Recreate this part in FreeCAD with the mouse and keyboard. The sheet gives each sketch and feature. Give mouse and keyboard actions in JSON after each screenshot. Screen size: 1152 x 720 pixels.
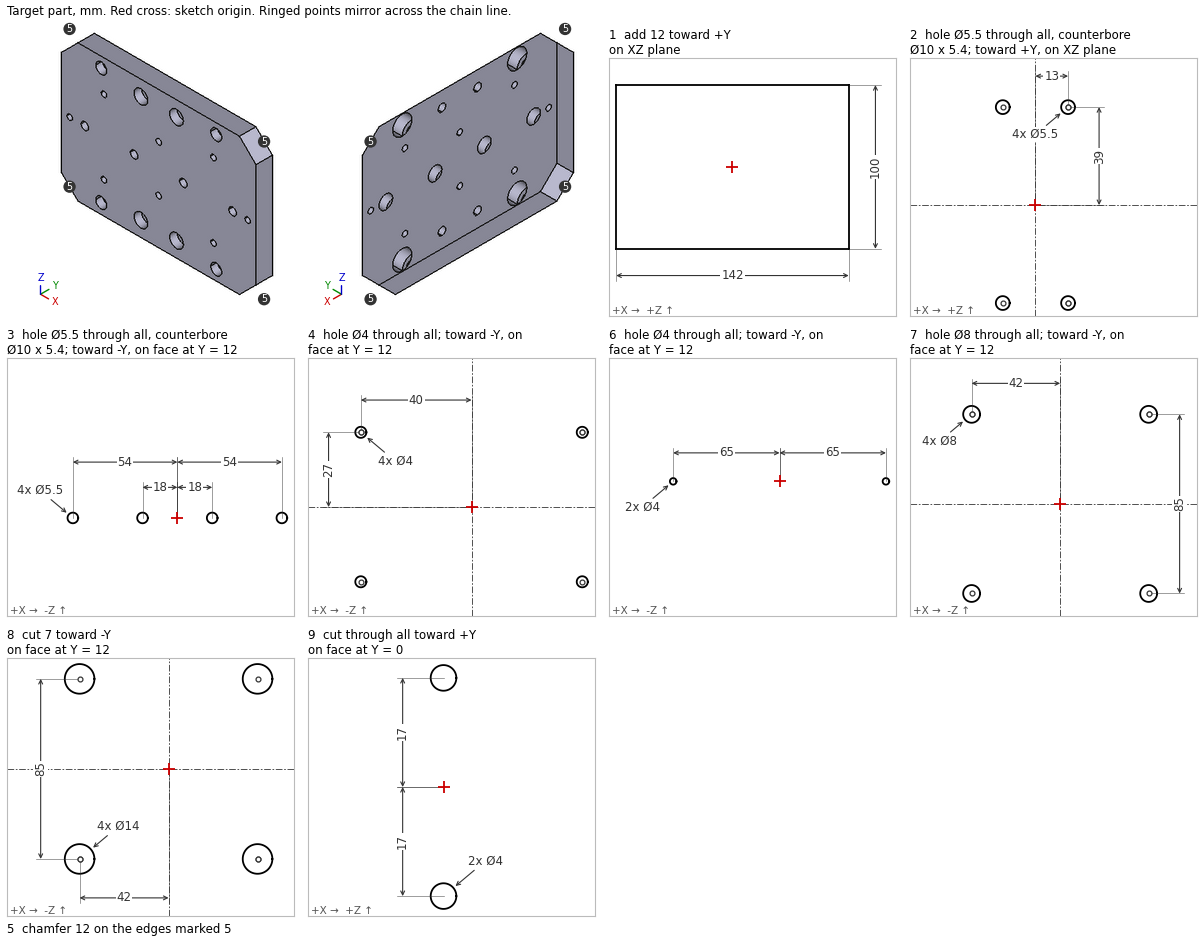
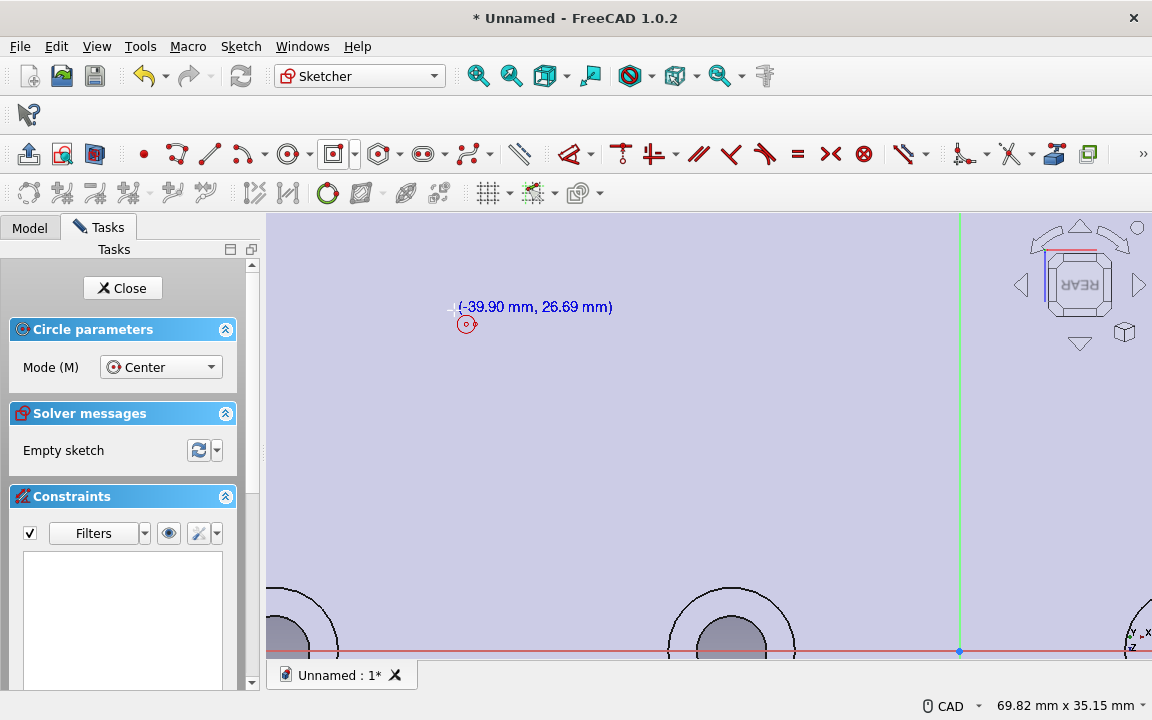
{"action": "left_click", "coordinate": [452, 308]}
{"action": "left_click", "coordinate": [470, 290]}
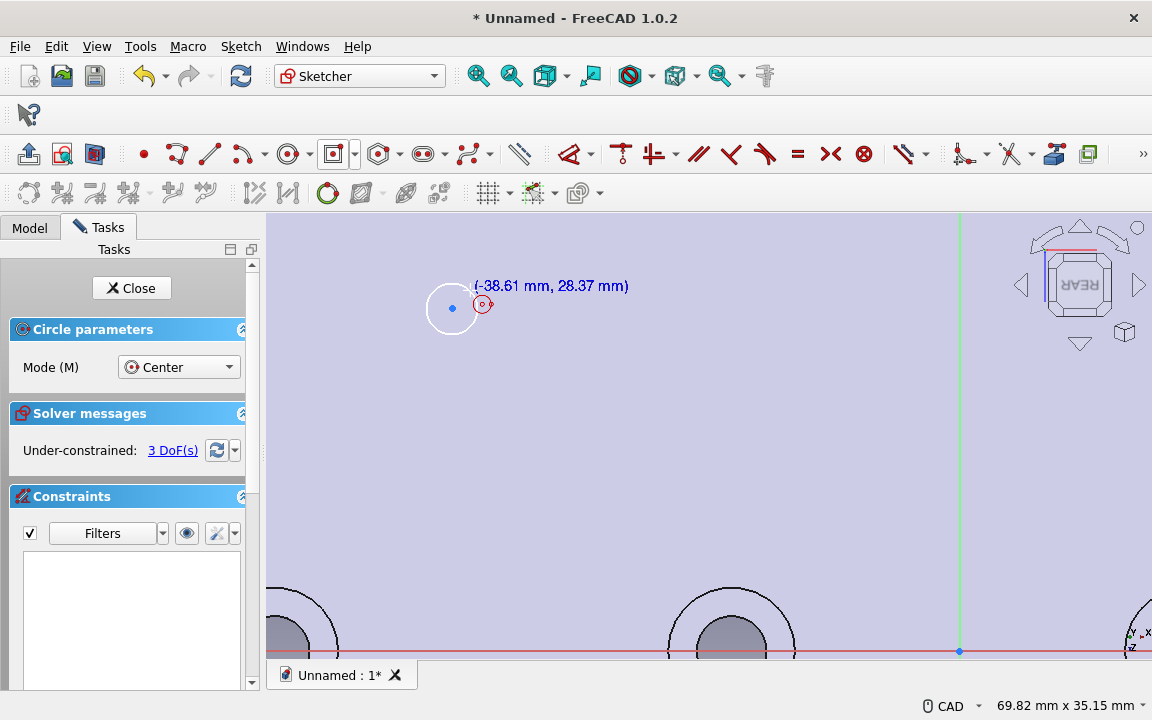
{"action": "scroll", "coordinate": [455, 311], "scroll_direction": "down", "scroll_amount": 5}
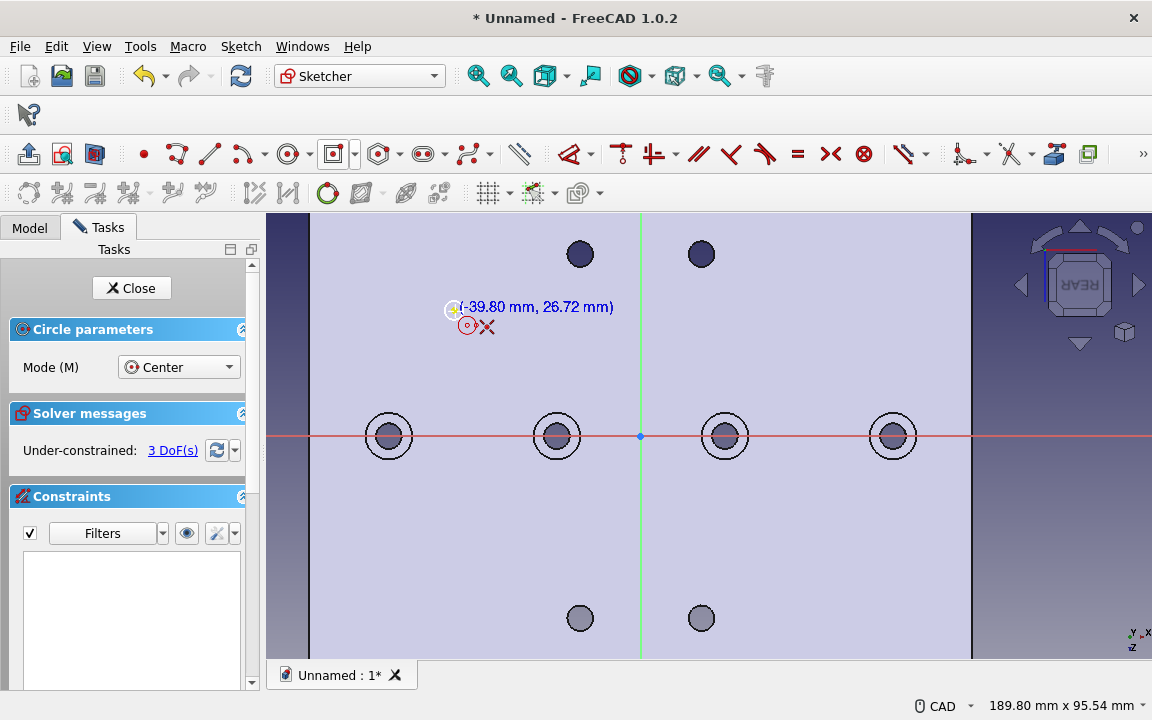
{"action": "scroll", "coordinate": [828, 310], "scroll_direction": "up", "scroll_amount": 5}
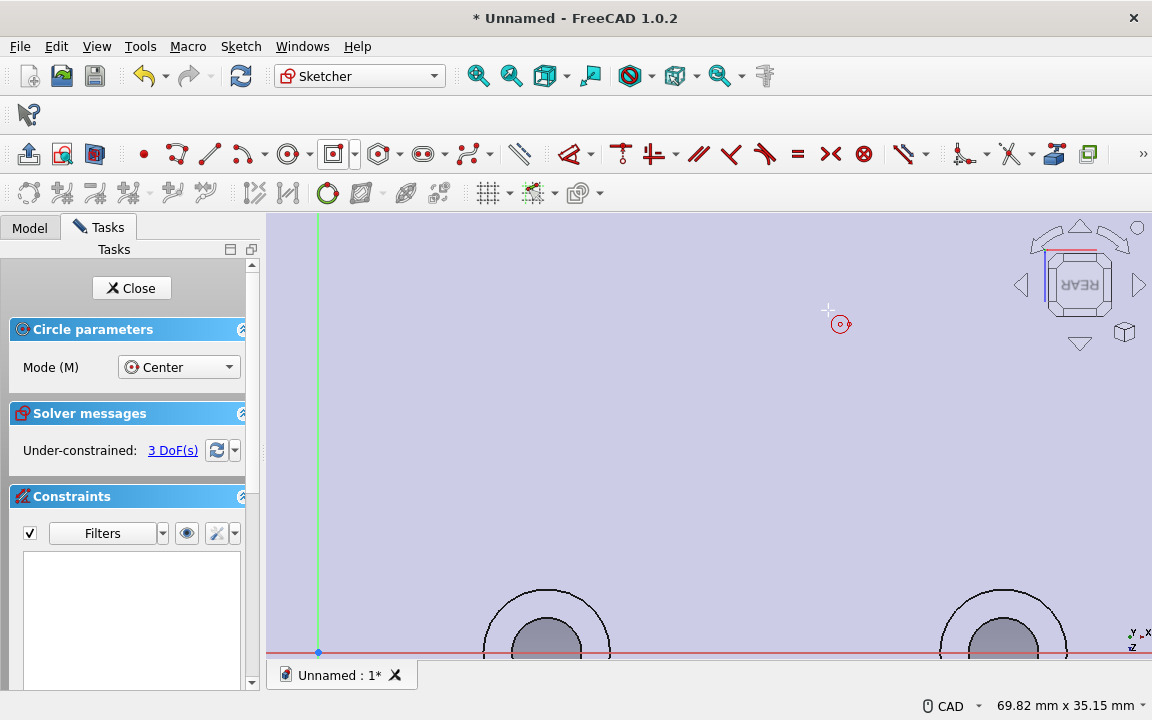
{"action": "left_click", "coordinate": [826, 310]}
{"action": "left_click", "coordinate": [844, 292]}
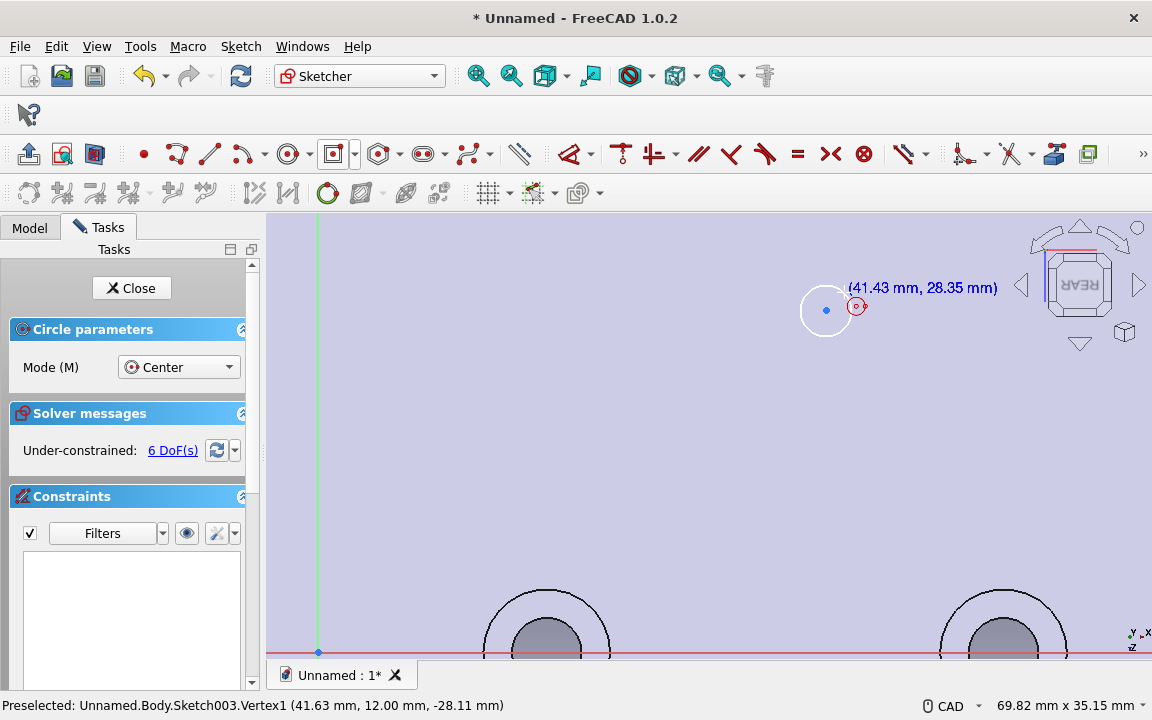
{"action": "scroll", "coordinate": [828, 310], "scroll_direction": "down", "scroll_amount": 5}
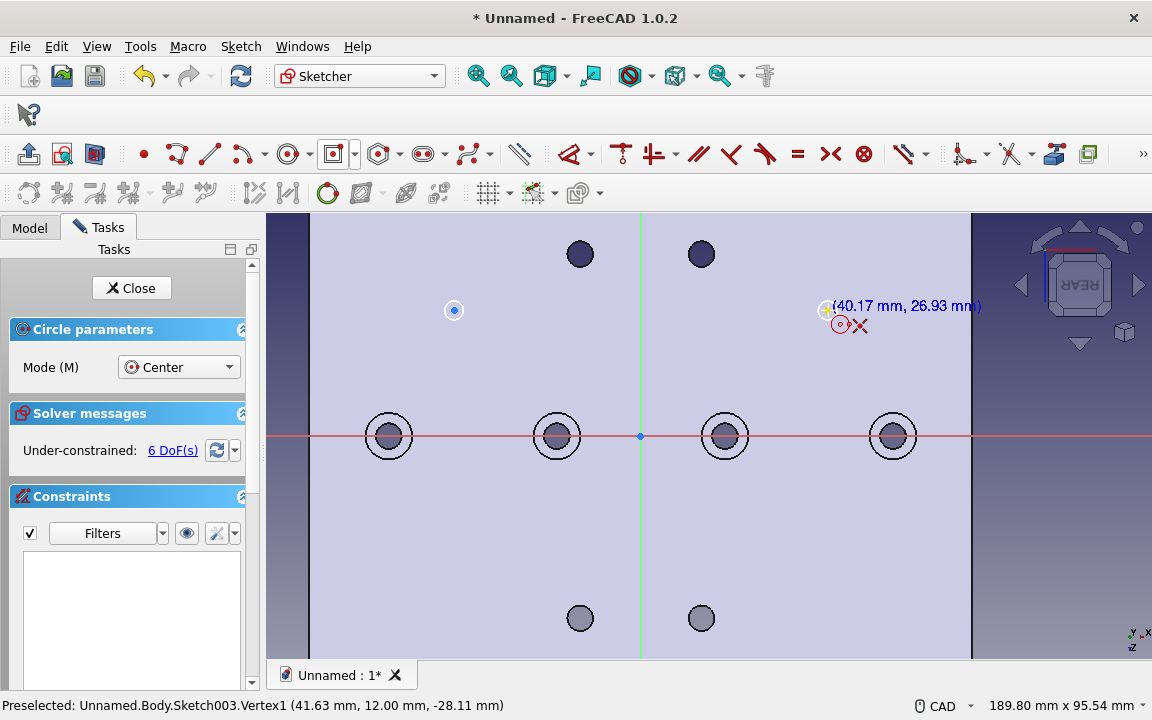
{"action": "scroll", "coordinate": [828, 562], "scroll_direction": "up", "scroll_amount": 5}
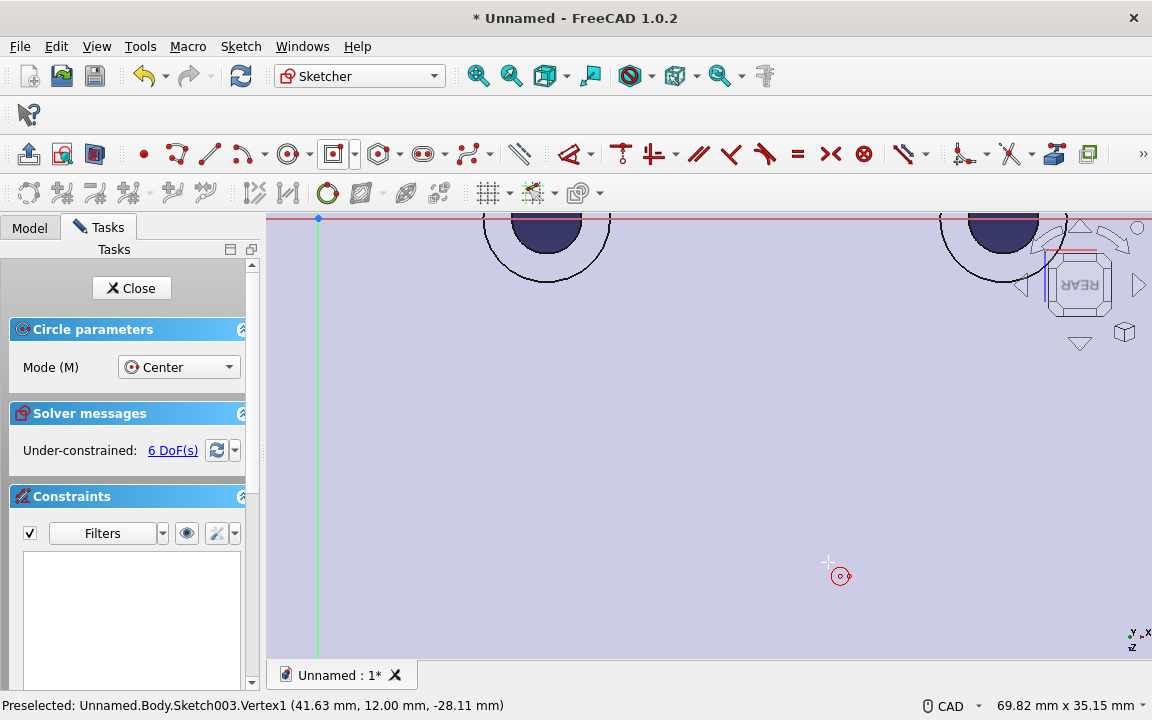
{"action": "left_click", "coordinate": [826, 561]}
{"action": "left_click", "coordinate": [844, 543]}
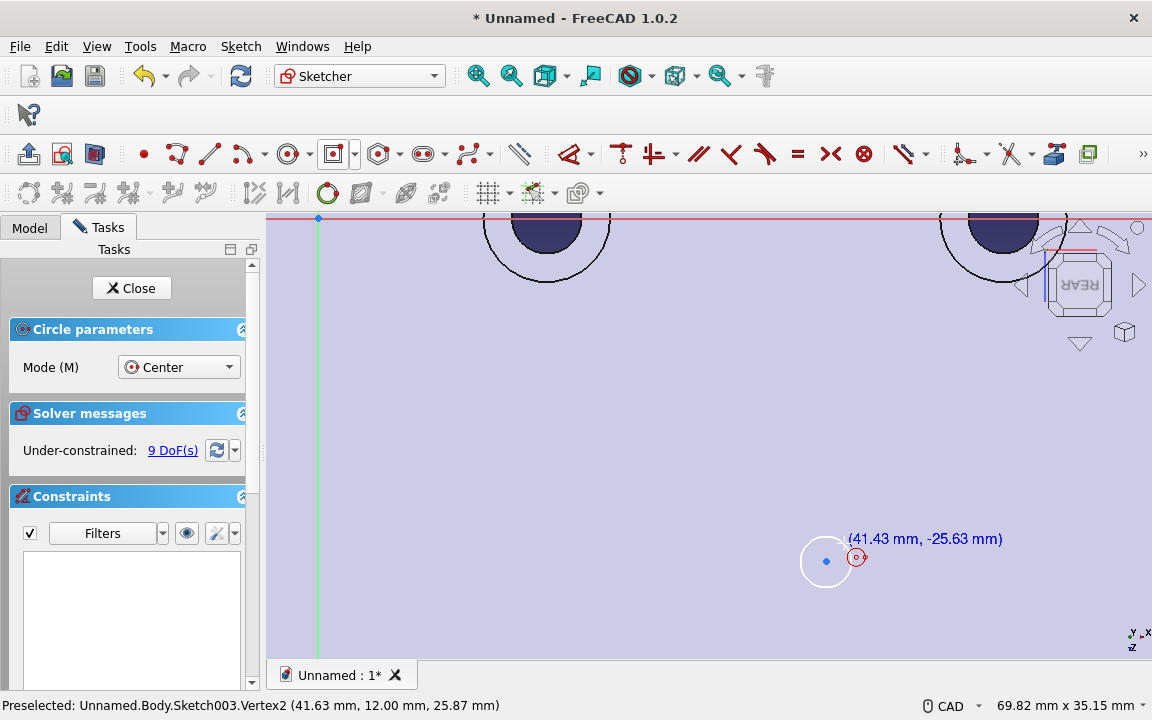
{"action": "scroll", "coordinate": [828, 562], "scroll_direction": "down", "scroll_amount": 5}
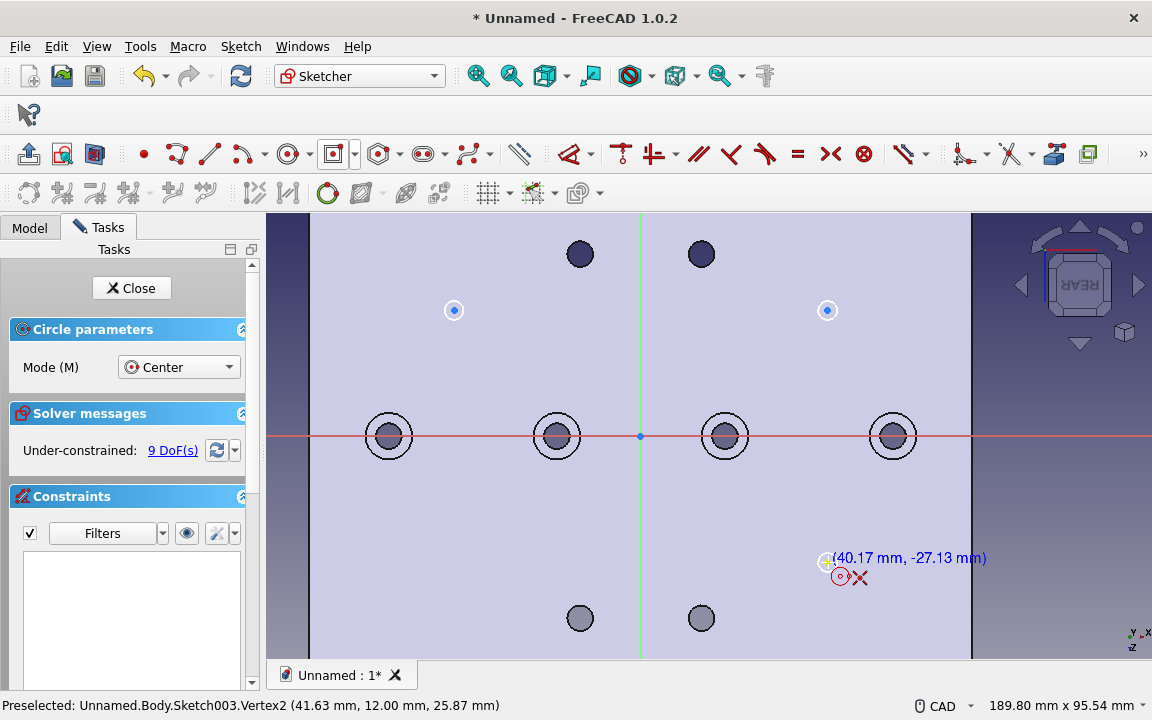
{"action": "scroll", "coordinate": [454, 562], "scroll_direction": "up", "scroll_amount": 5}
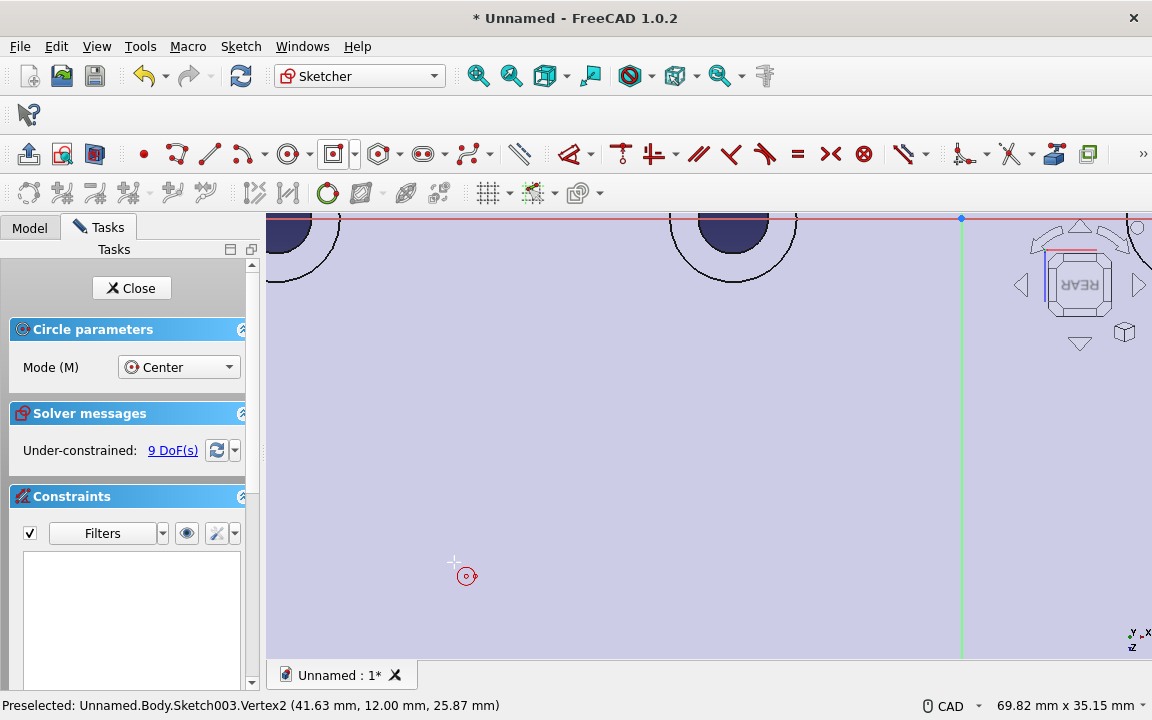
{"action": "left_click", "coordinate": [454, 561]}
{"action": "left_click", "coordinate": [472, 543]}
{"action": "key", "text": "Escape"}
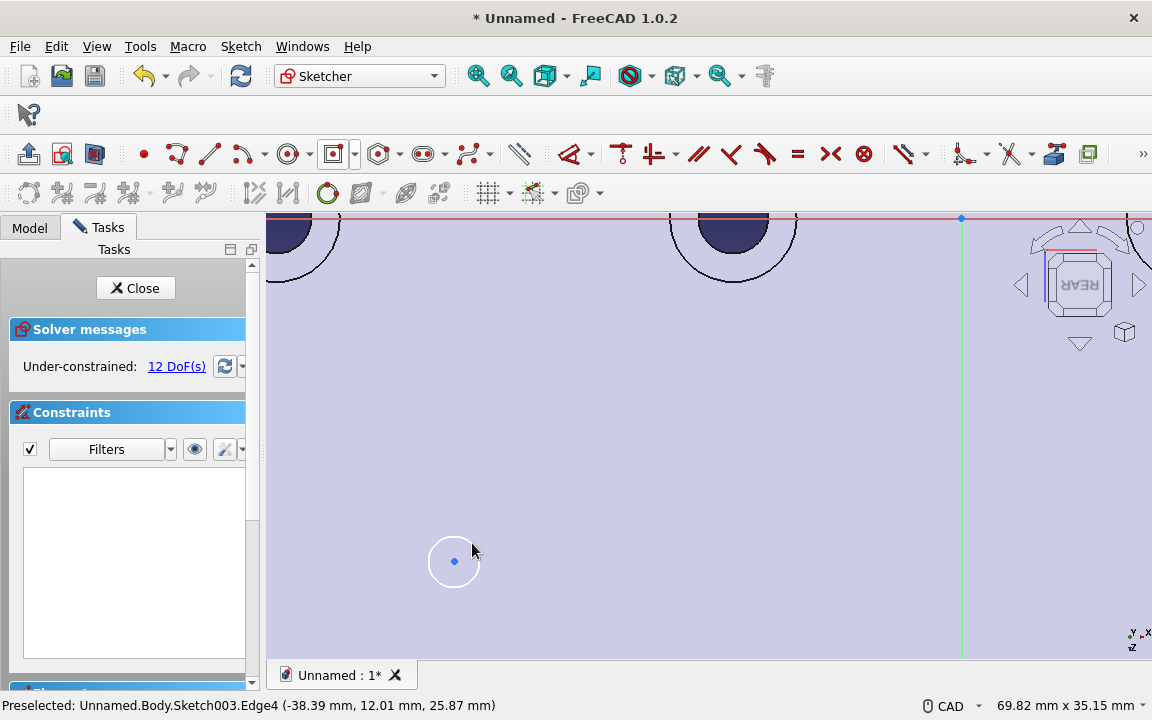
{"action": "scroll", "coordinate": [454, 562], "scroll_direction": "down", "scroll_amount": 5}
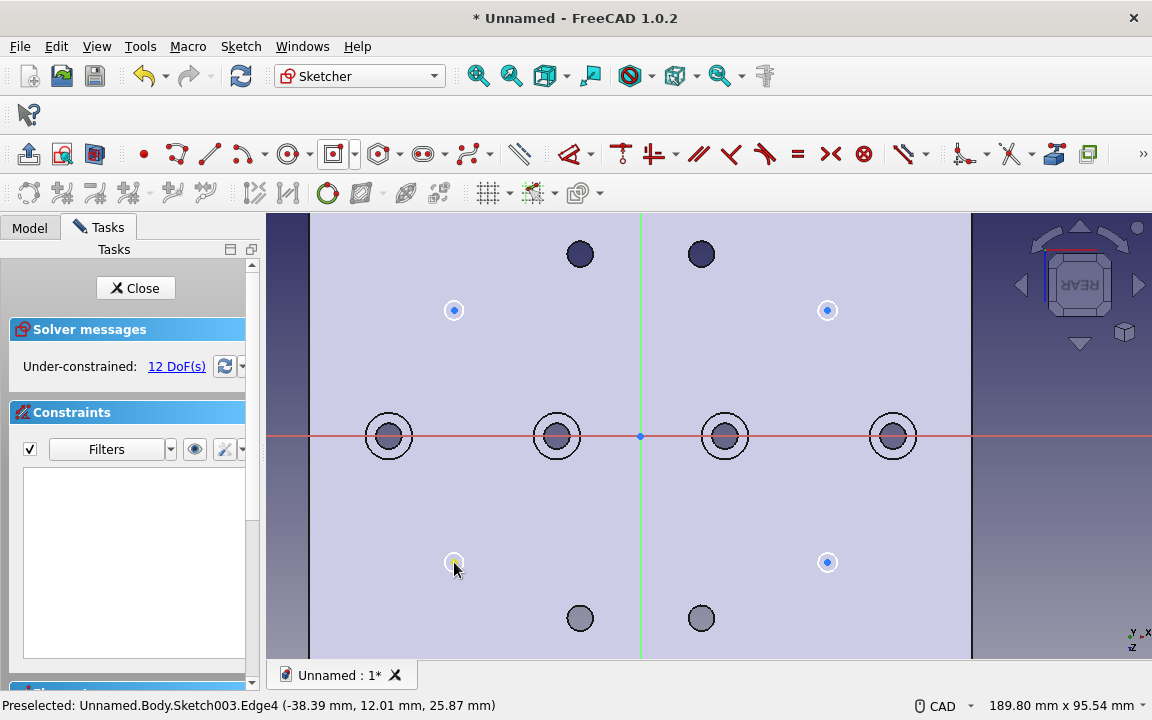
{"action": "scroll", "coordinate": [461, 304], "scroll_direction": "up", "scroll_amount": 2}